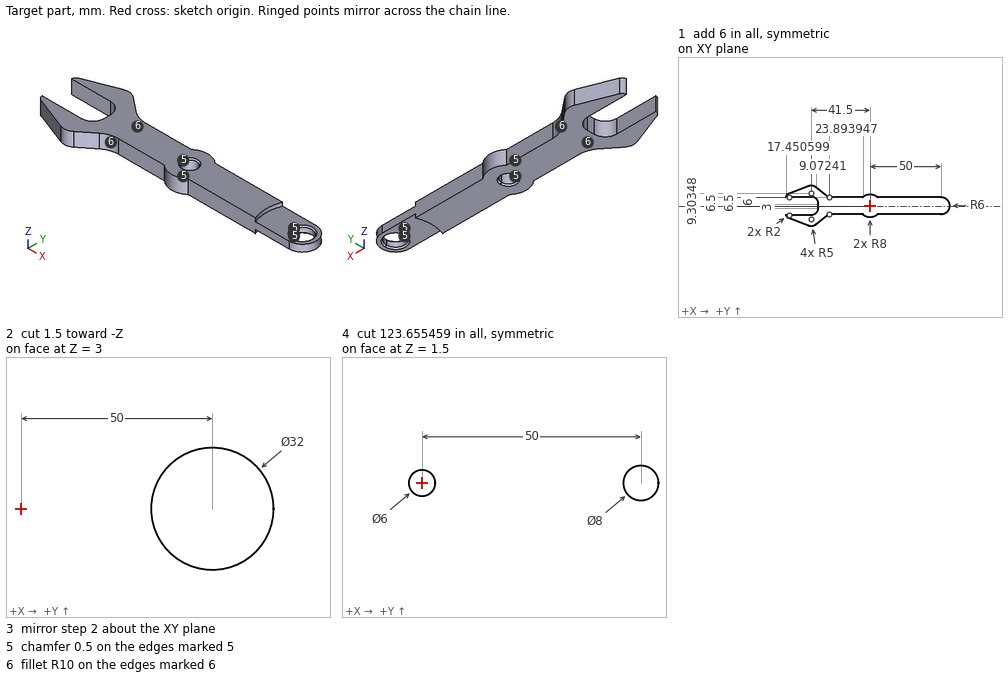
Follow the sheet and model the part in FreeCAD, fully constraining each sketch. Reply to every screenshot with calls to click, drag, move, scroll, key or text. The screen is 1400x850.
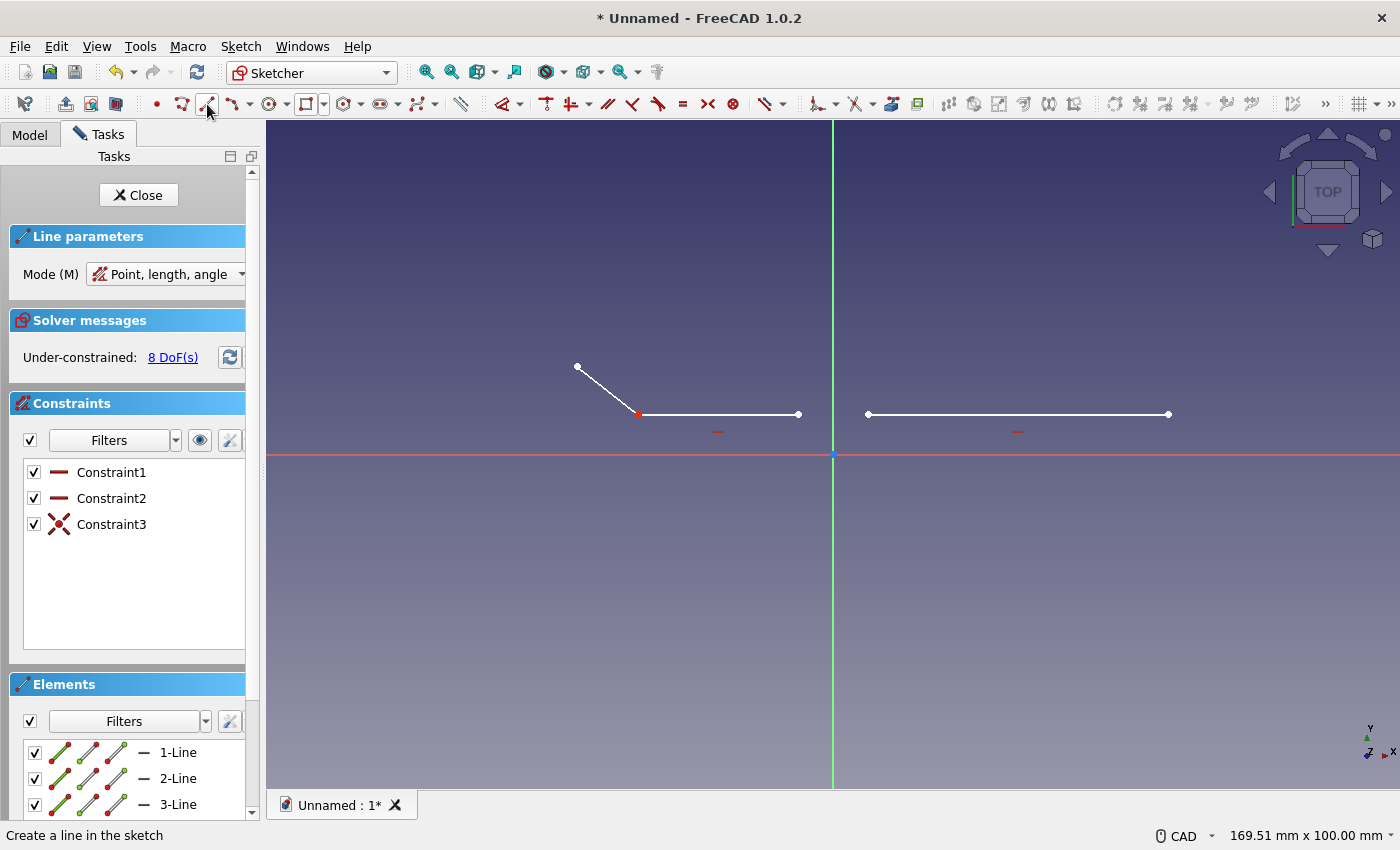
click(544, 361)
click(447, 399)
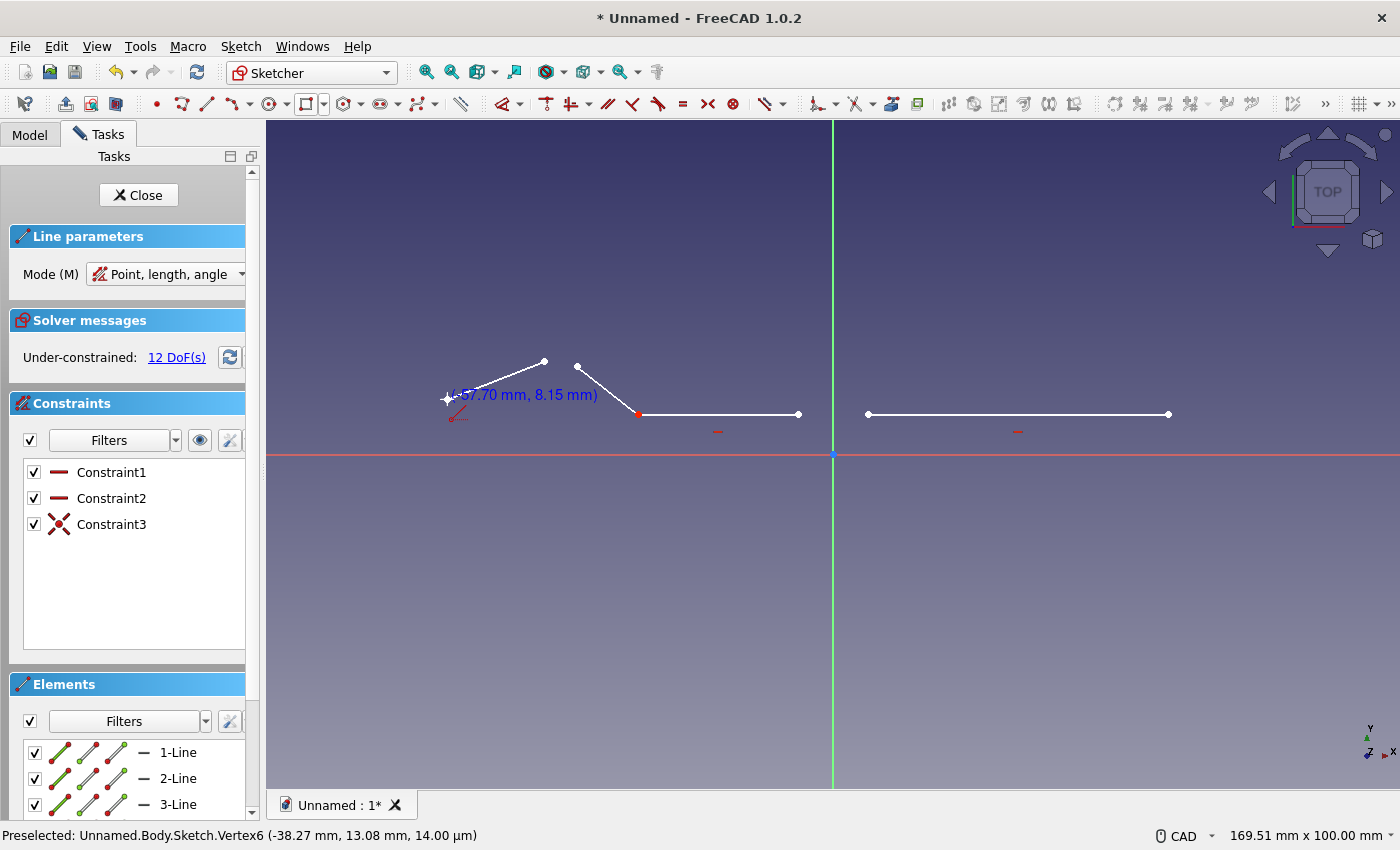
click(439, 411)
click(555, 411)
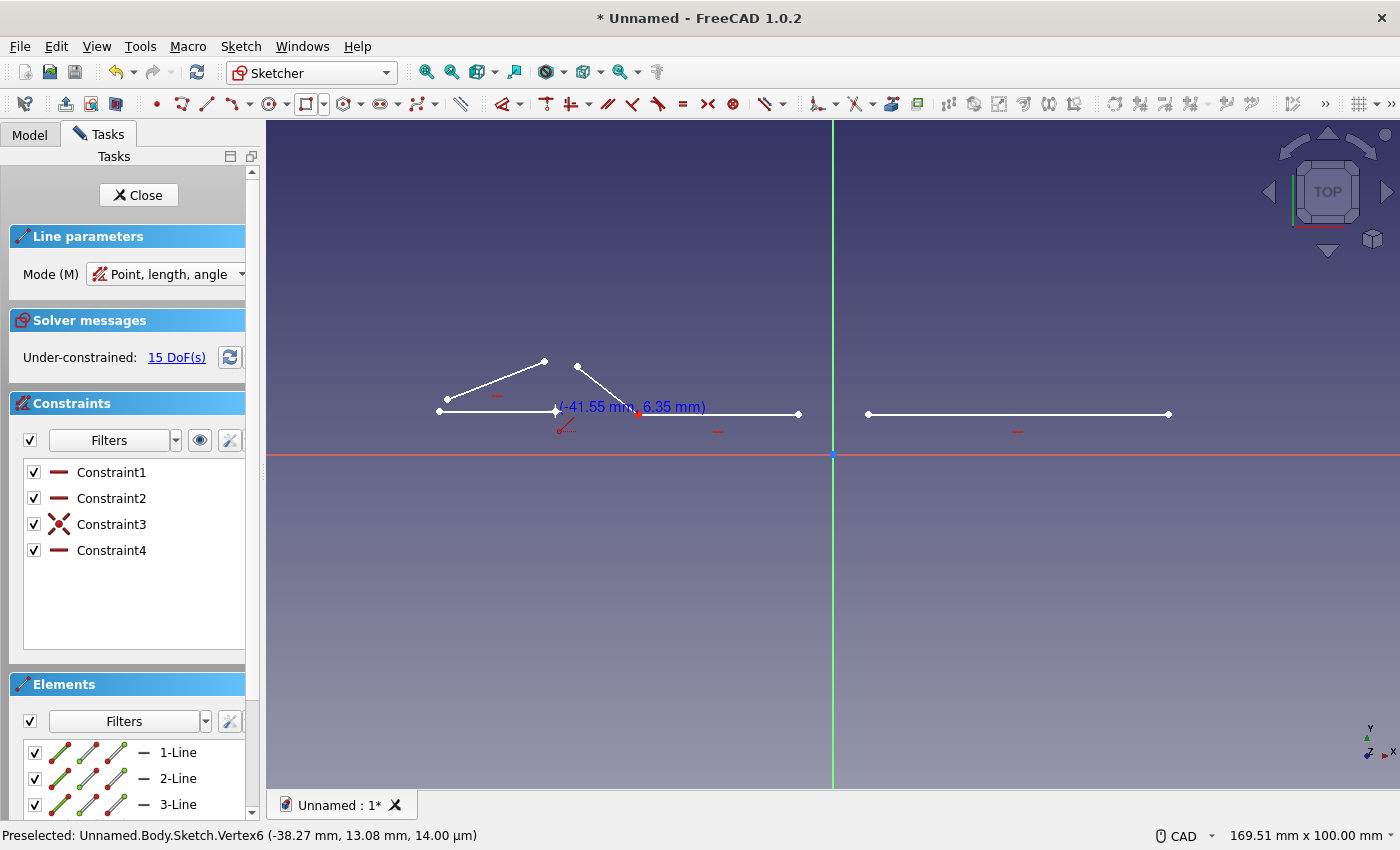
scroll(589, 444, up, 3)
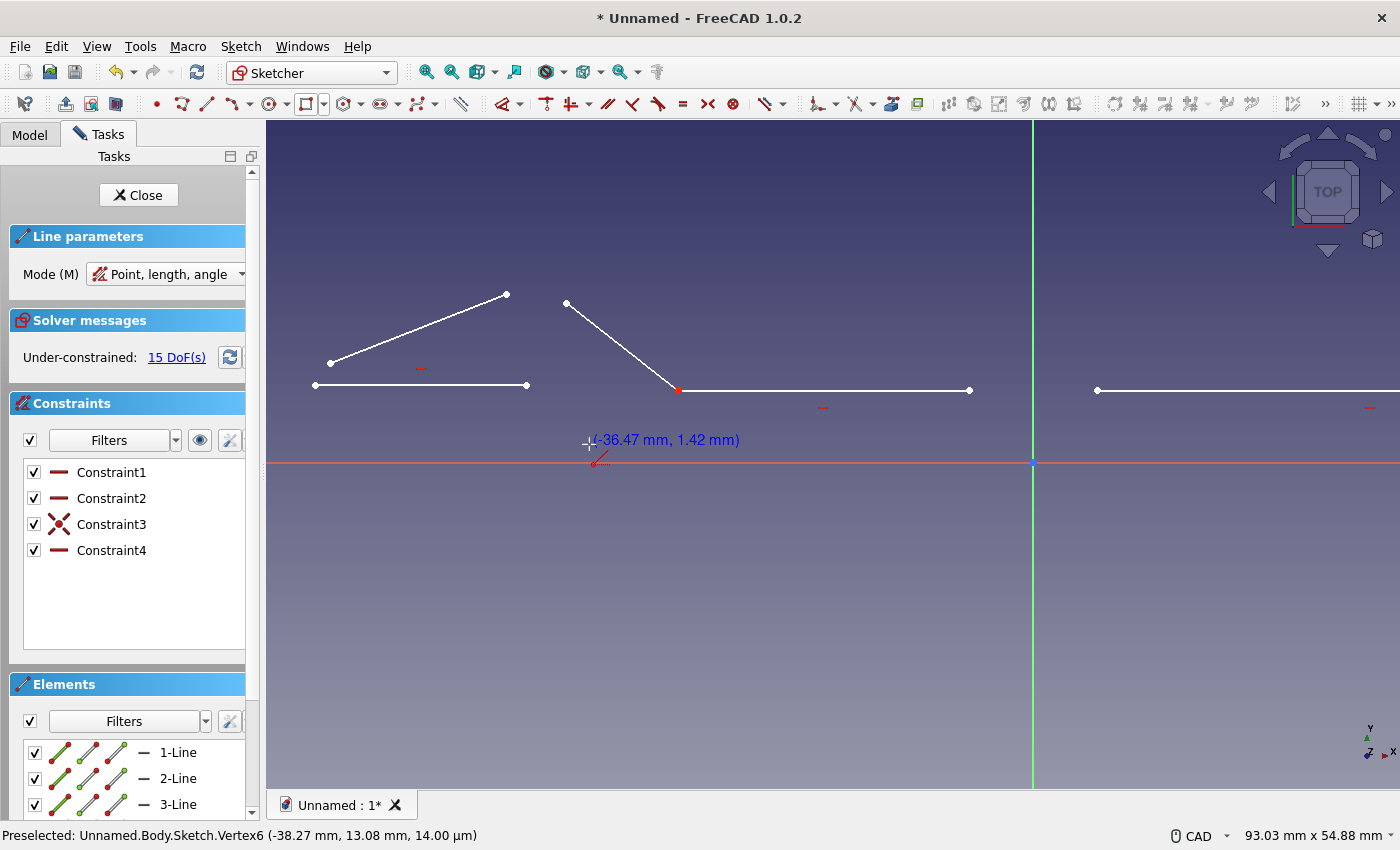
click(588, 444)
click(588, 481)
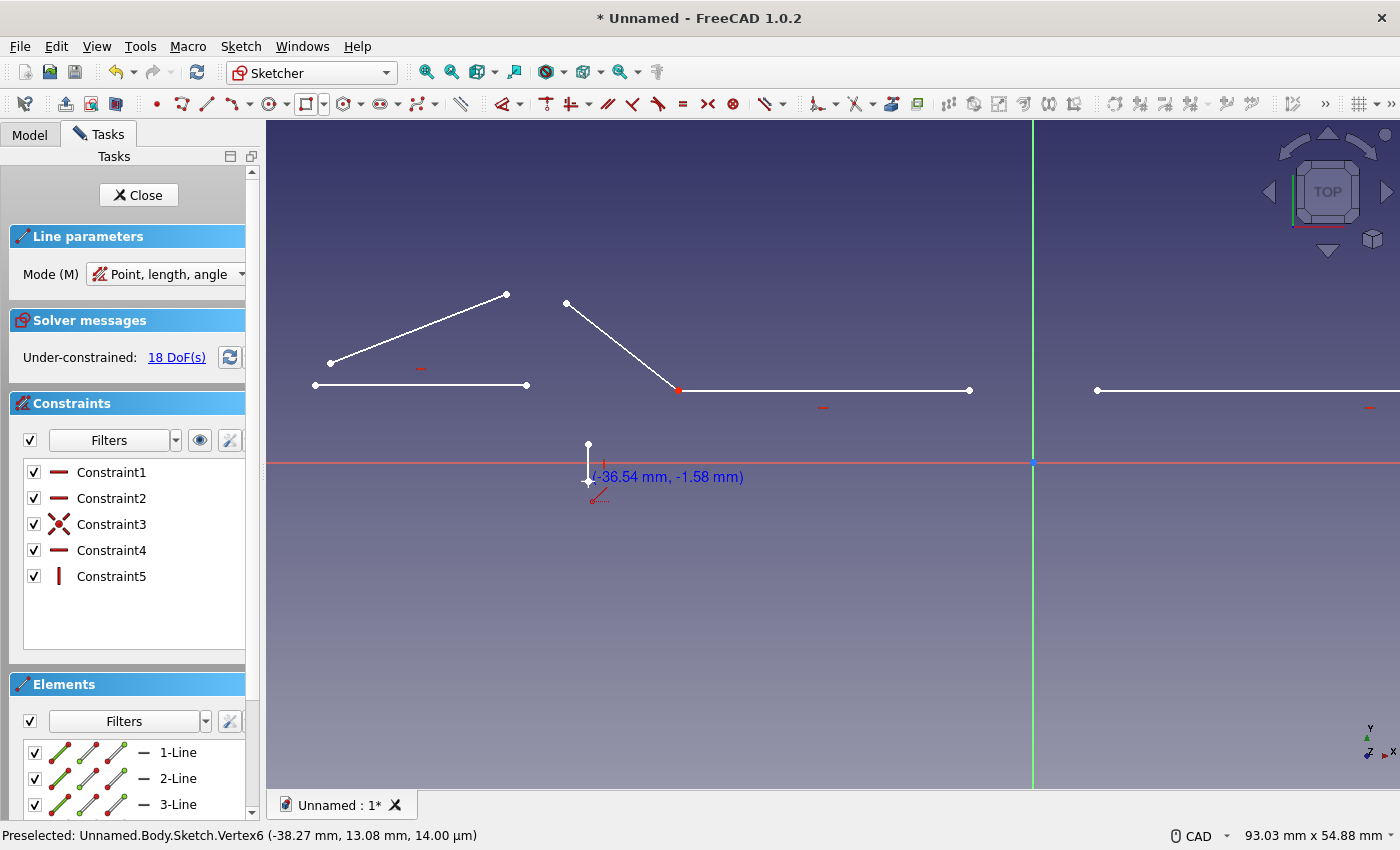
click(527, 542)
click(315, 542)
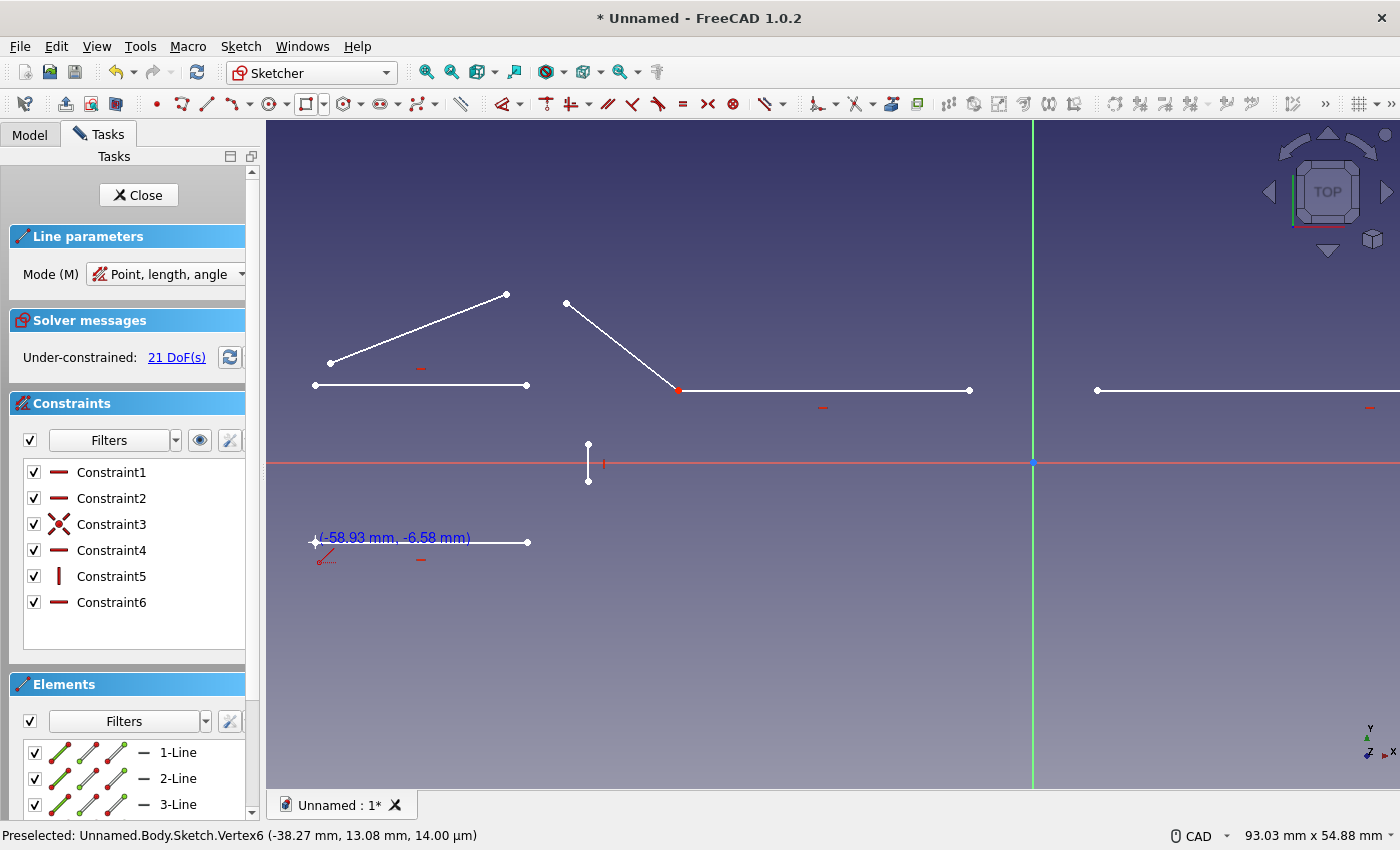
click(330, 565)
click(507, 633)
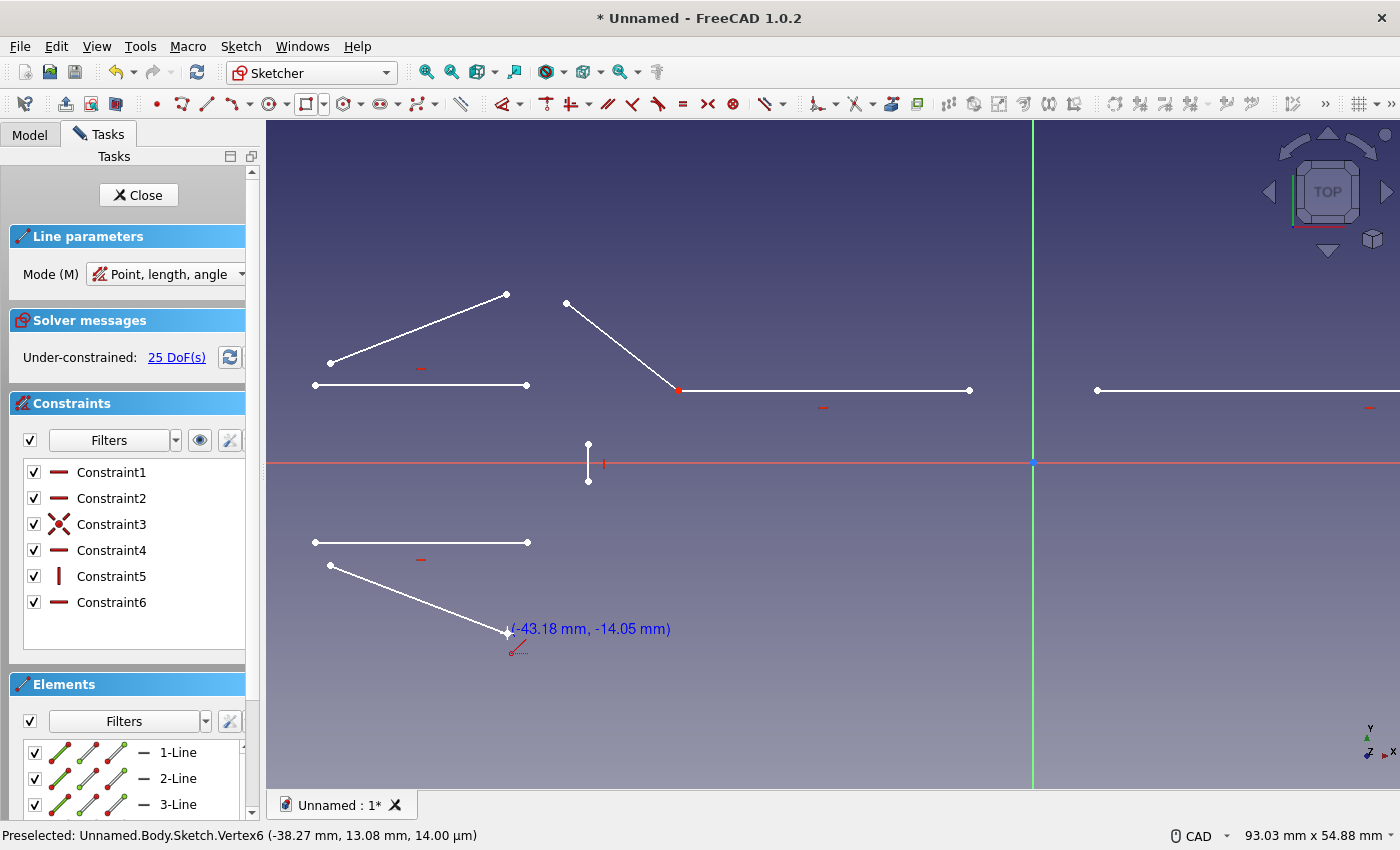
click(182, 104)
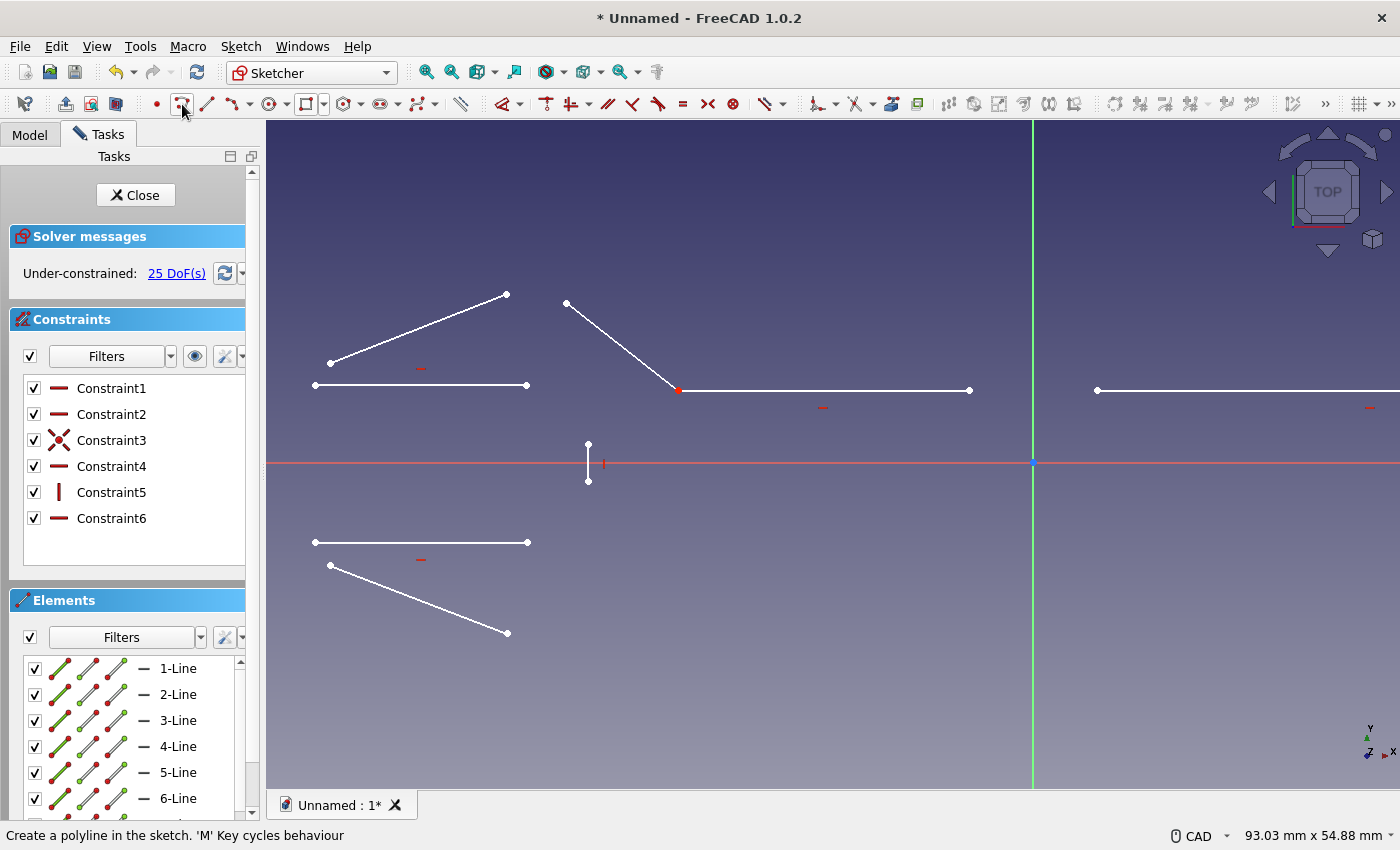
click(567, 624)
click(678, 536)
click(969, 536)
right_click(969, 536)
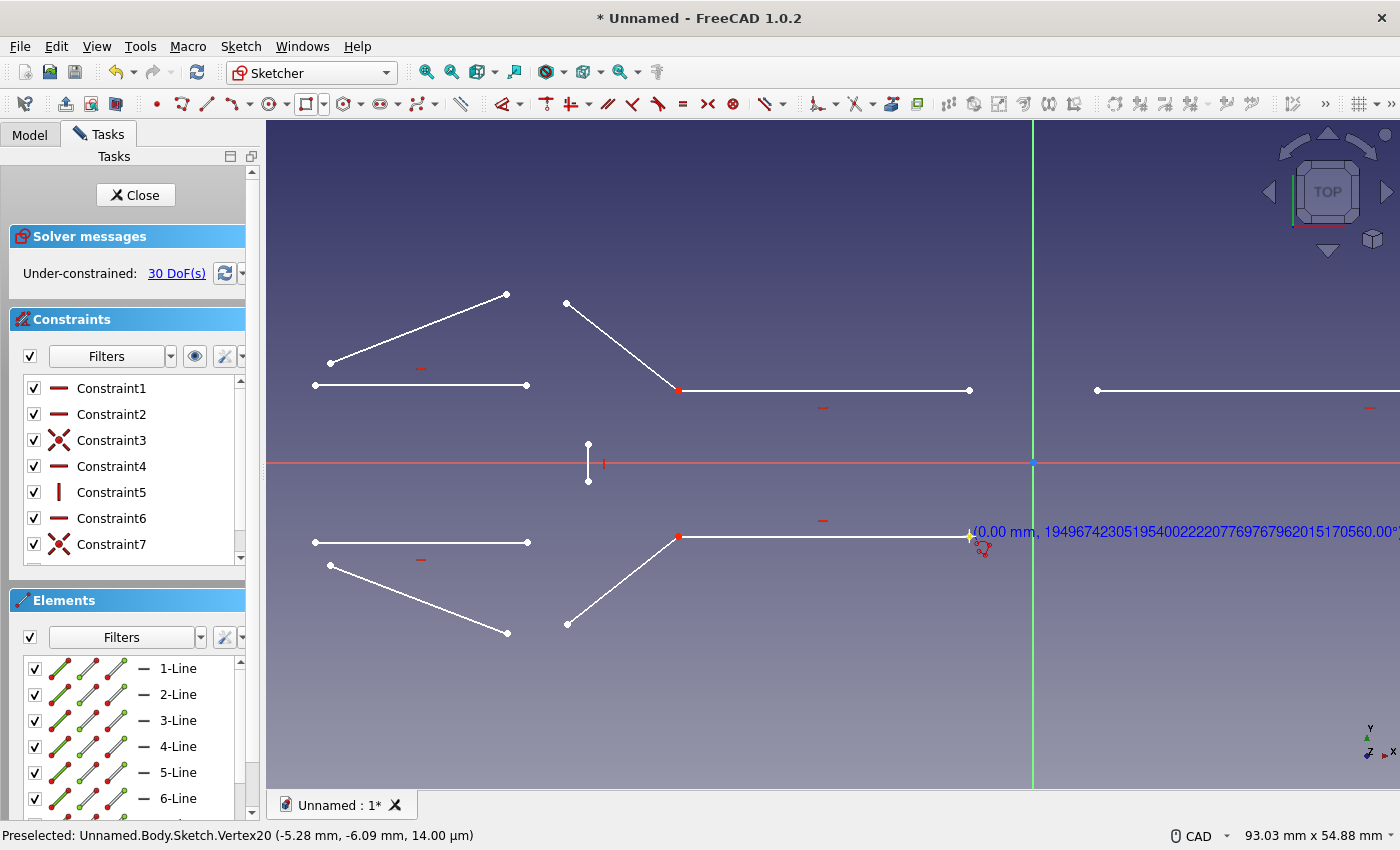
click(207, 104)